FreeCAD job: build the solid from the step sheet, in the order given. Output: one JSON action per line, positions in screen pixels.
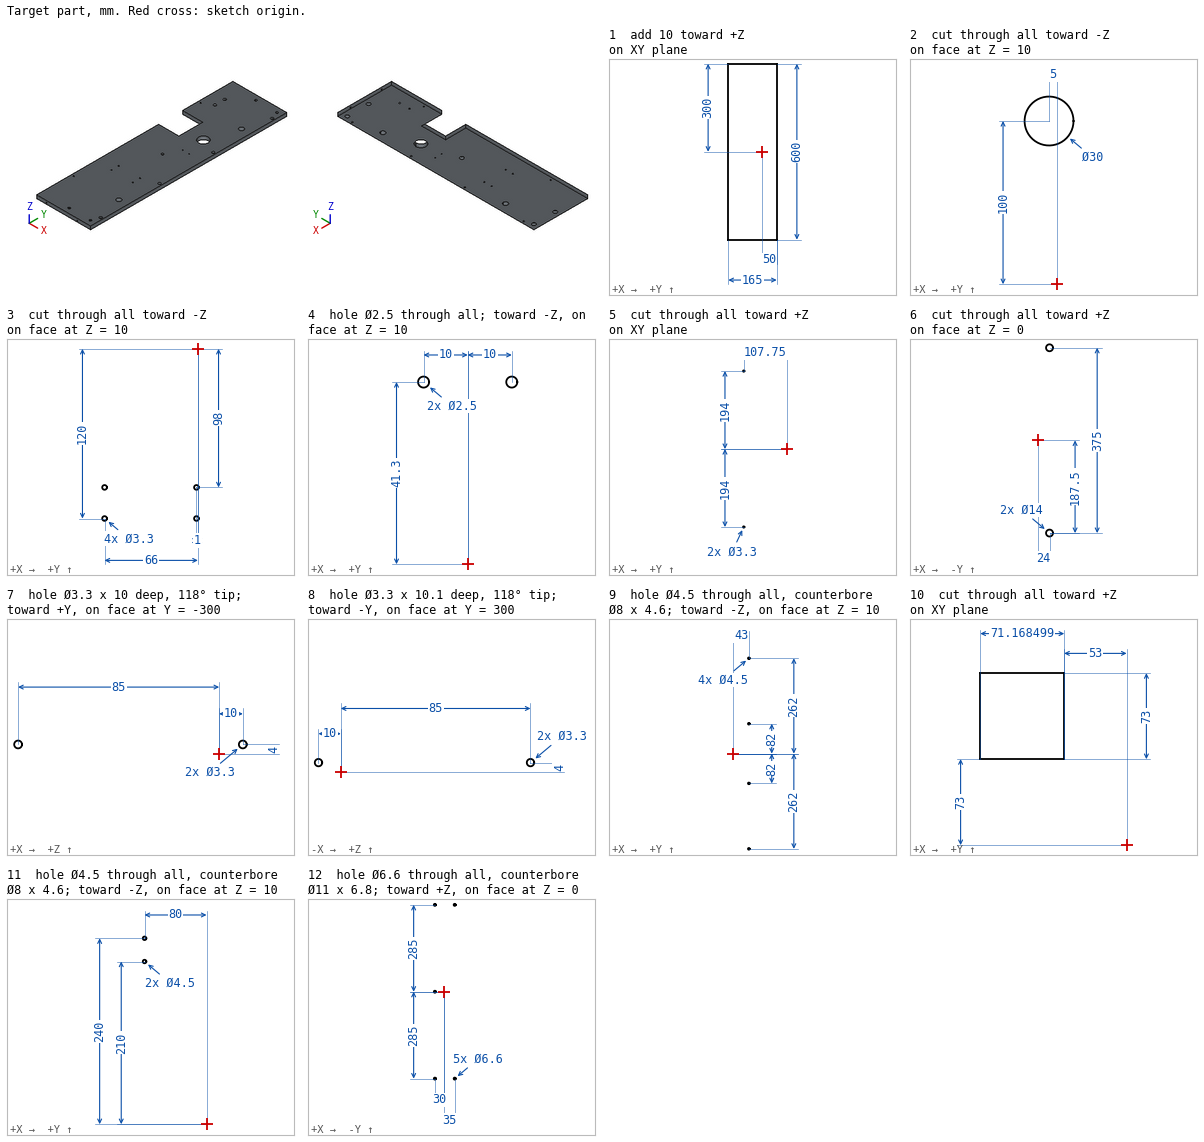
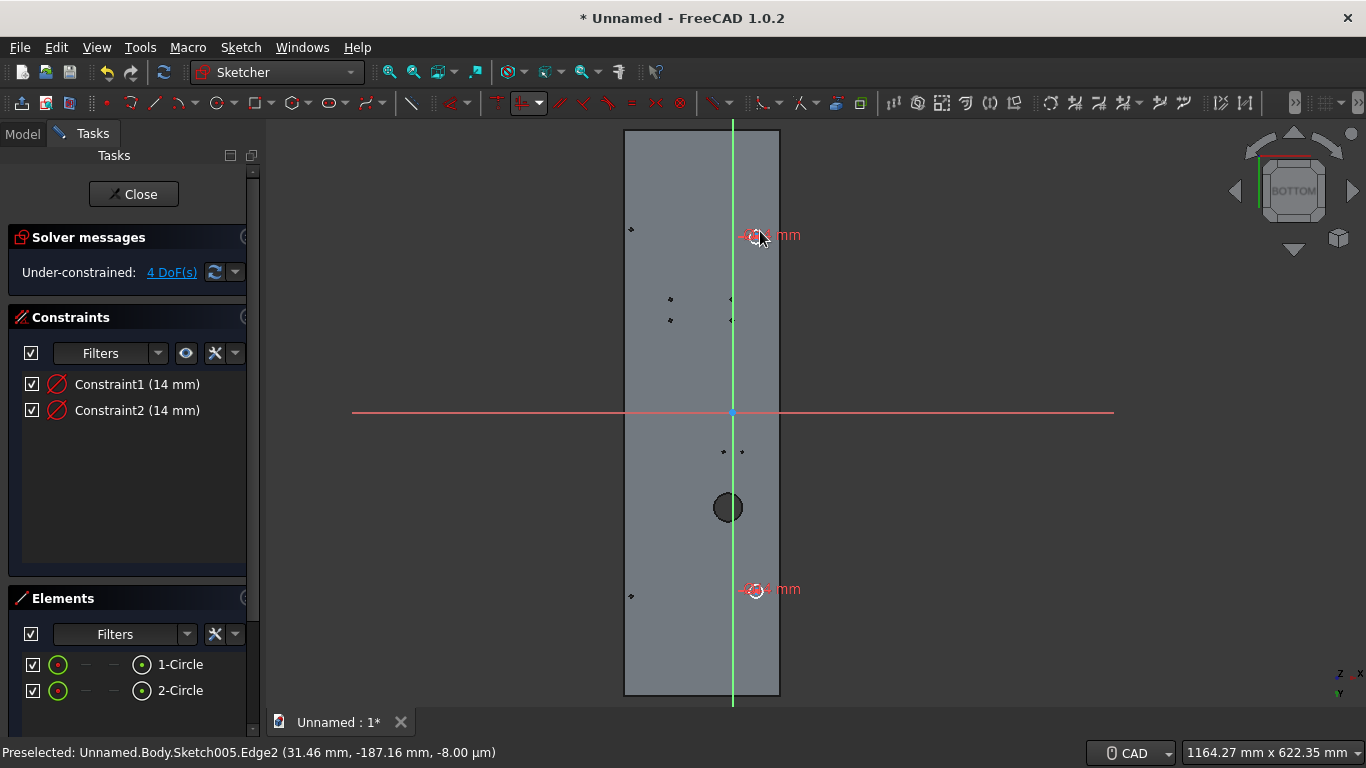
{"action": "left_click", "coordinate": [756, 591]}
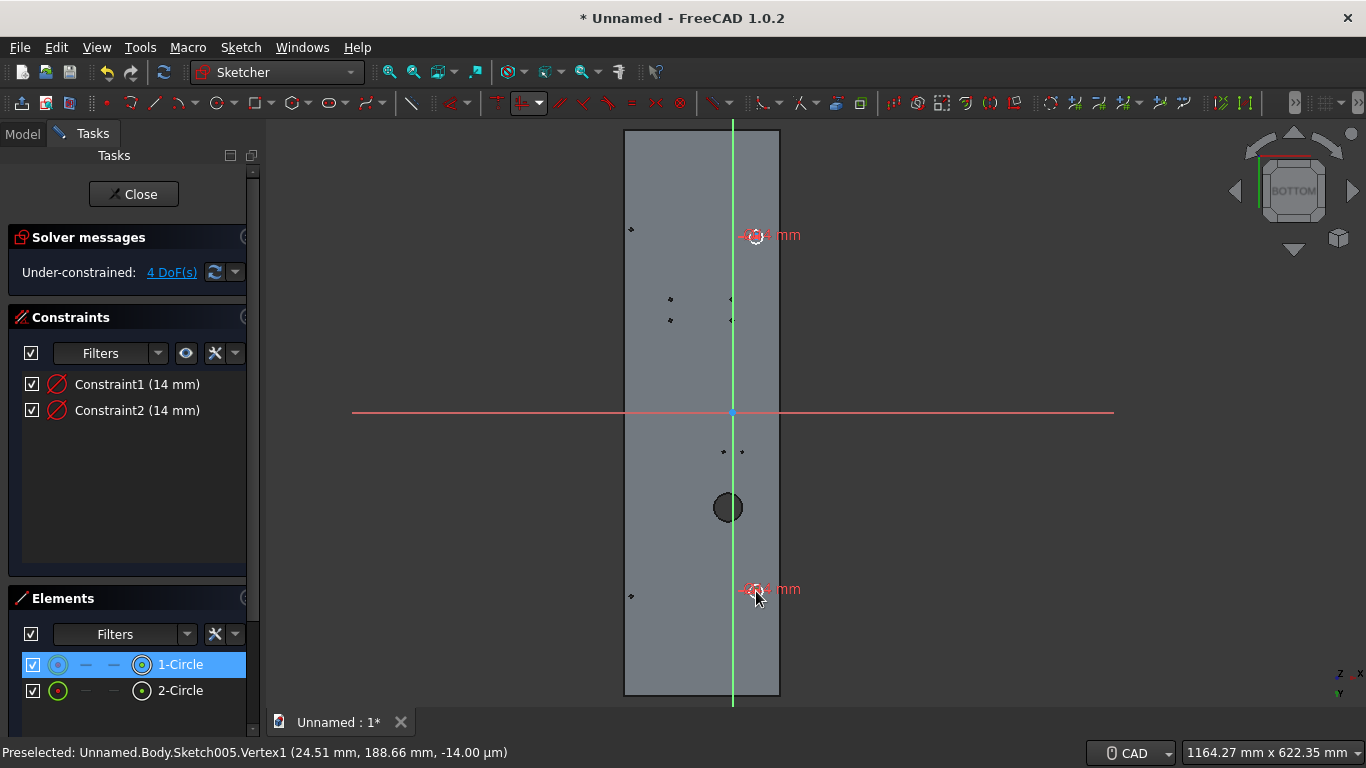
{"action": "left_click", "coordinate": [756, 237]}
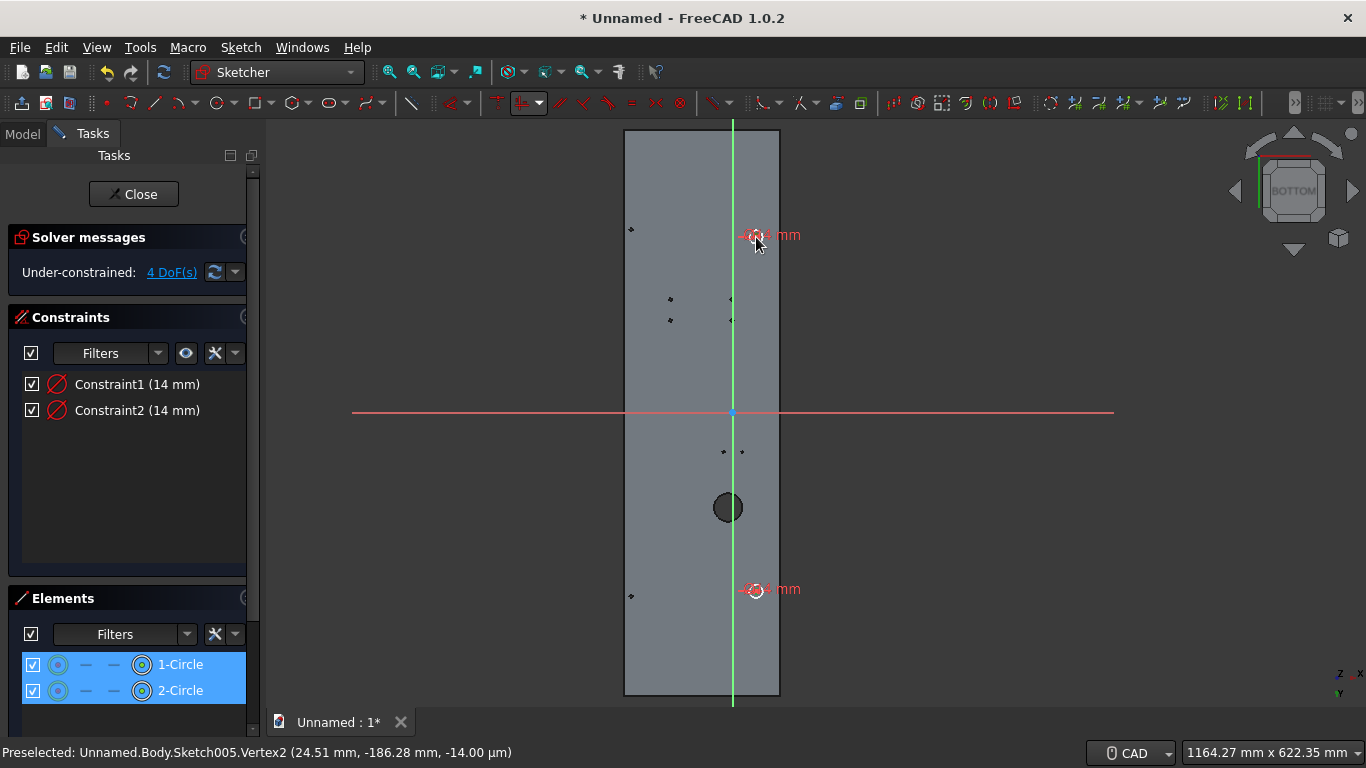
{"action": "key", "text": "v"}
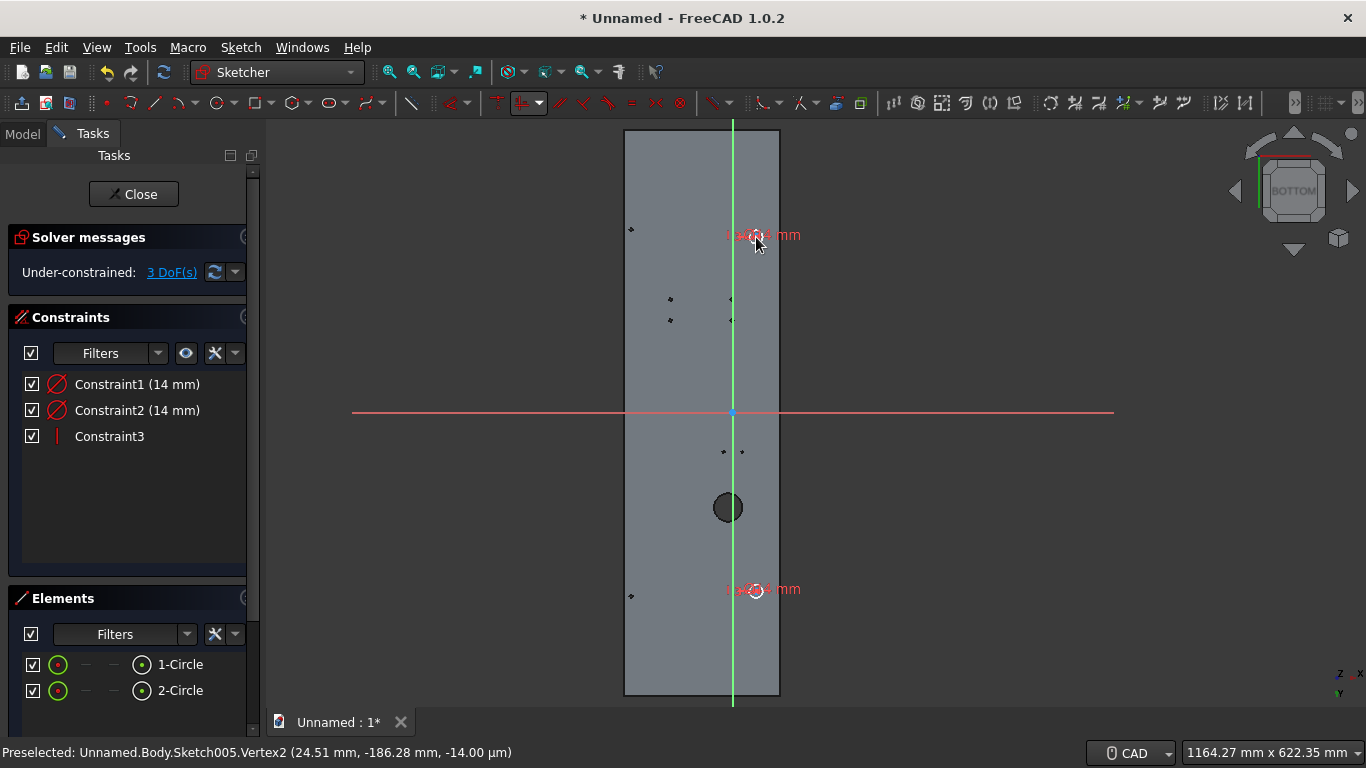
{"action": "key", "text": "d"}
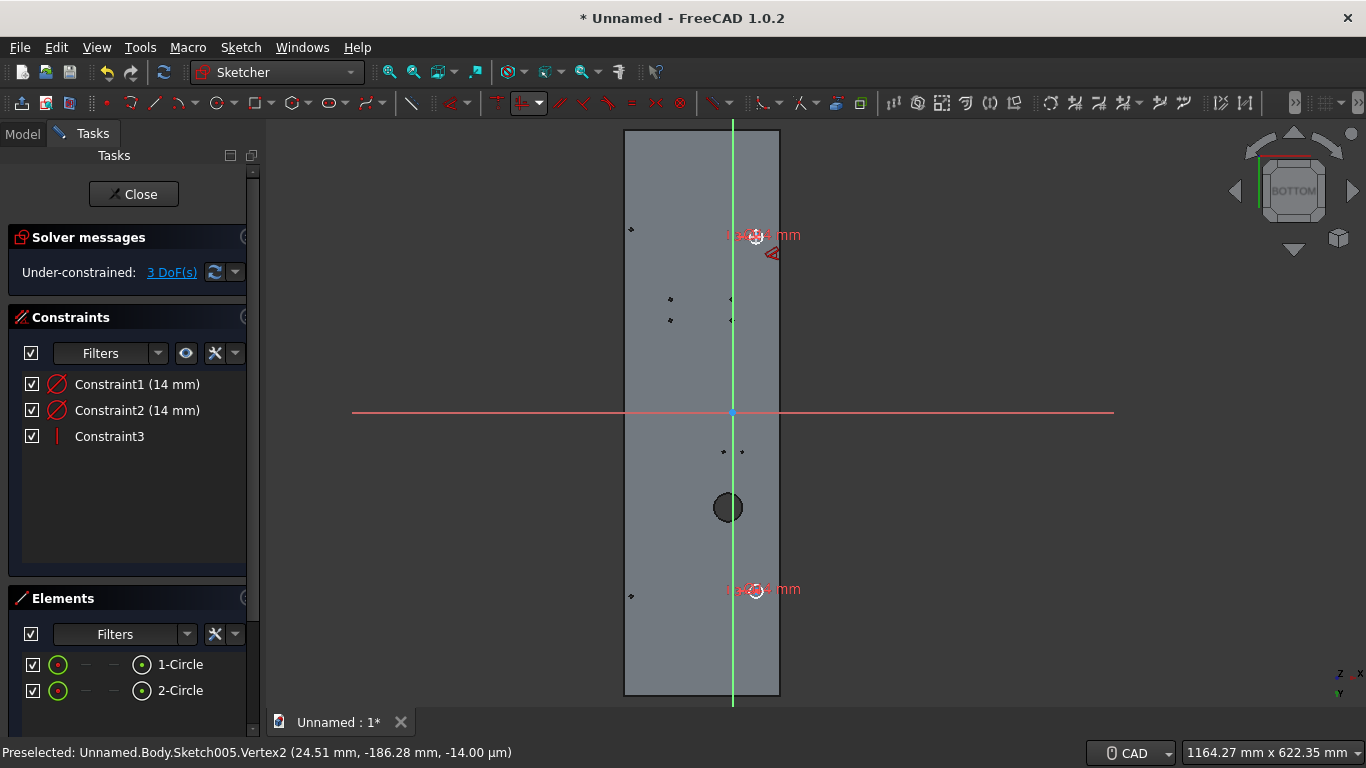
{"action": "scroll", "coordinate": [756, 591], "scroll_direction": "up", "scroll_amount": 3}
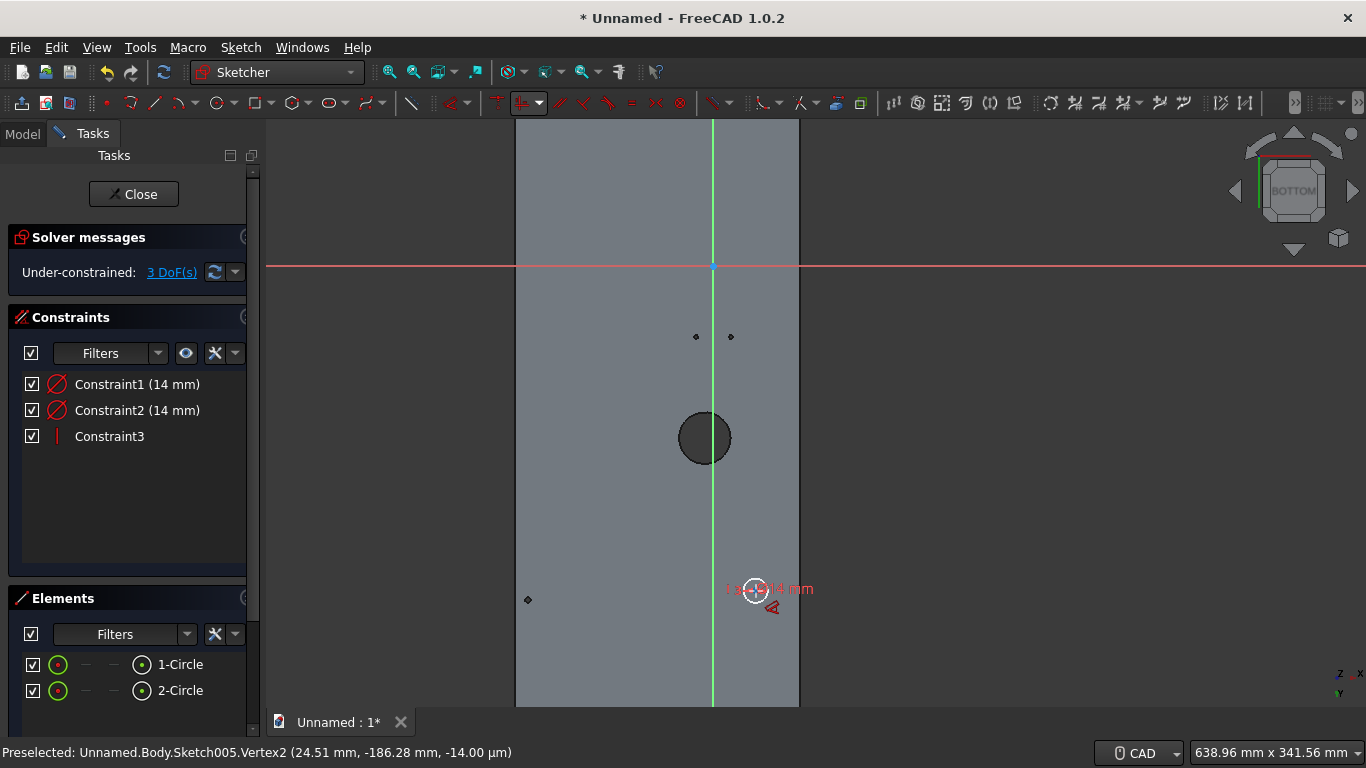
{"action": "left_click", "coordinate": [756, 591]}
{"action": "left_click", "coordinate": [735, 625]}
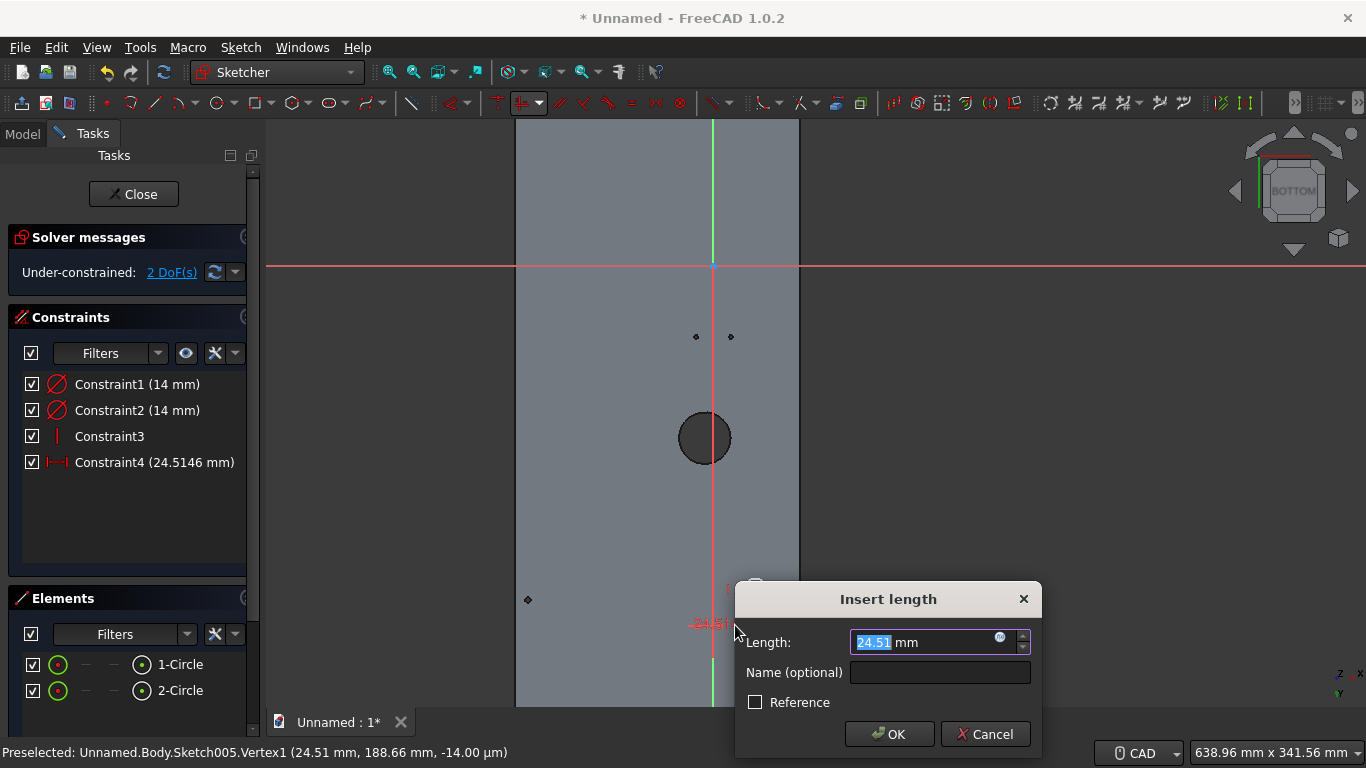
{"action": "type", "text": "24"}
{"action": "key", "text": "Return"}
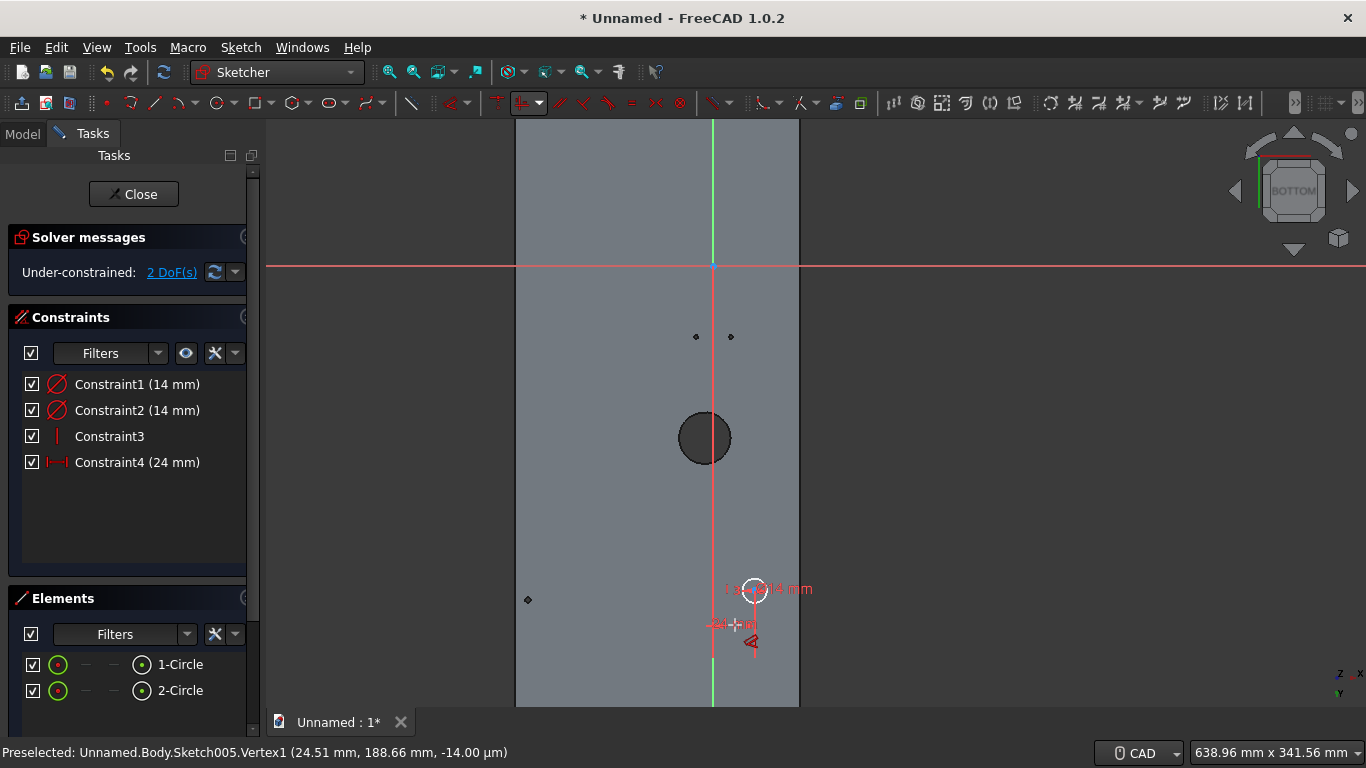
{"action": "left_click", "coordinate": [755, 591]}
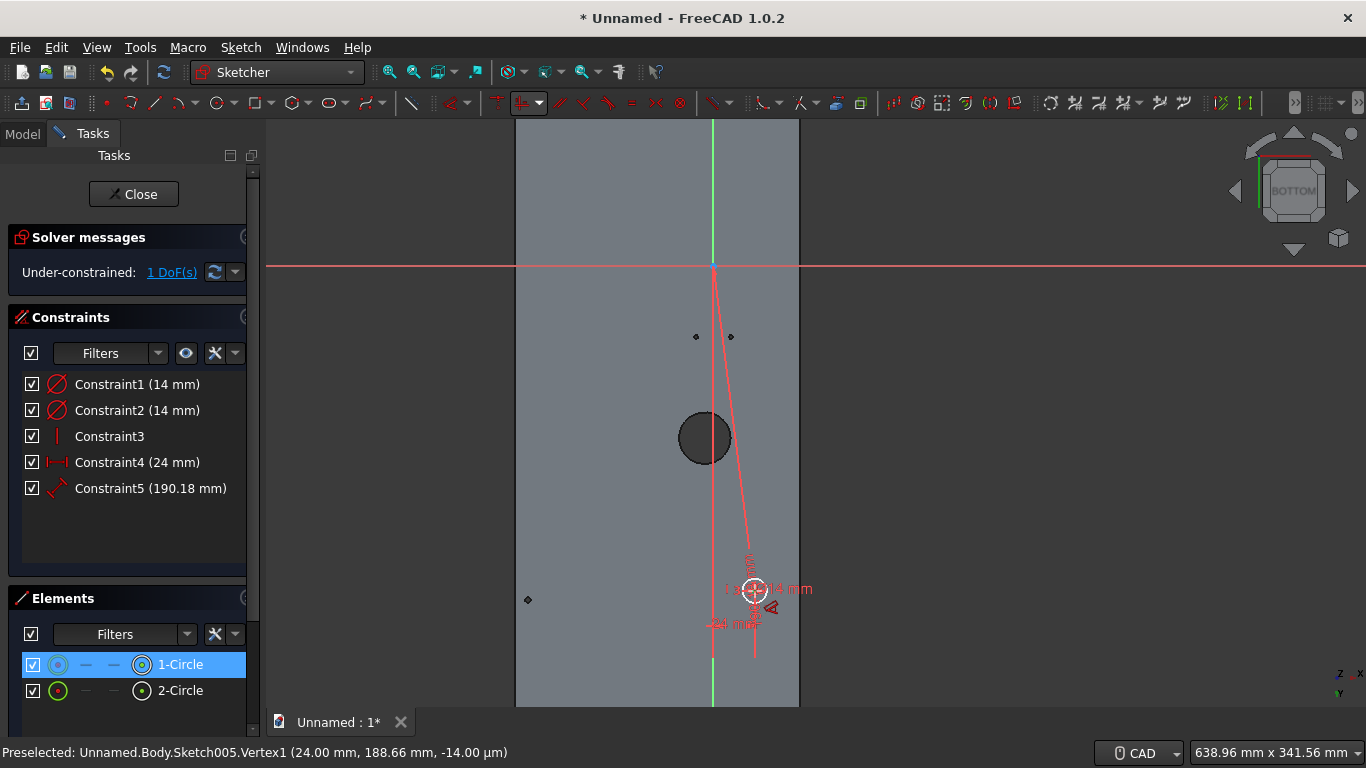
{"action": "scroll", "coordinate": [756, 592], "scroll_direction": "down", "scroll_amount": 3}